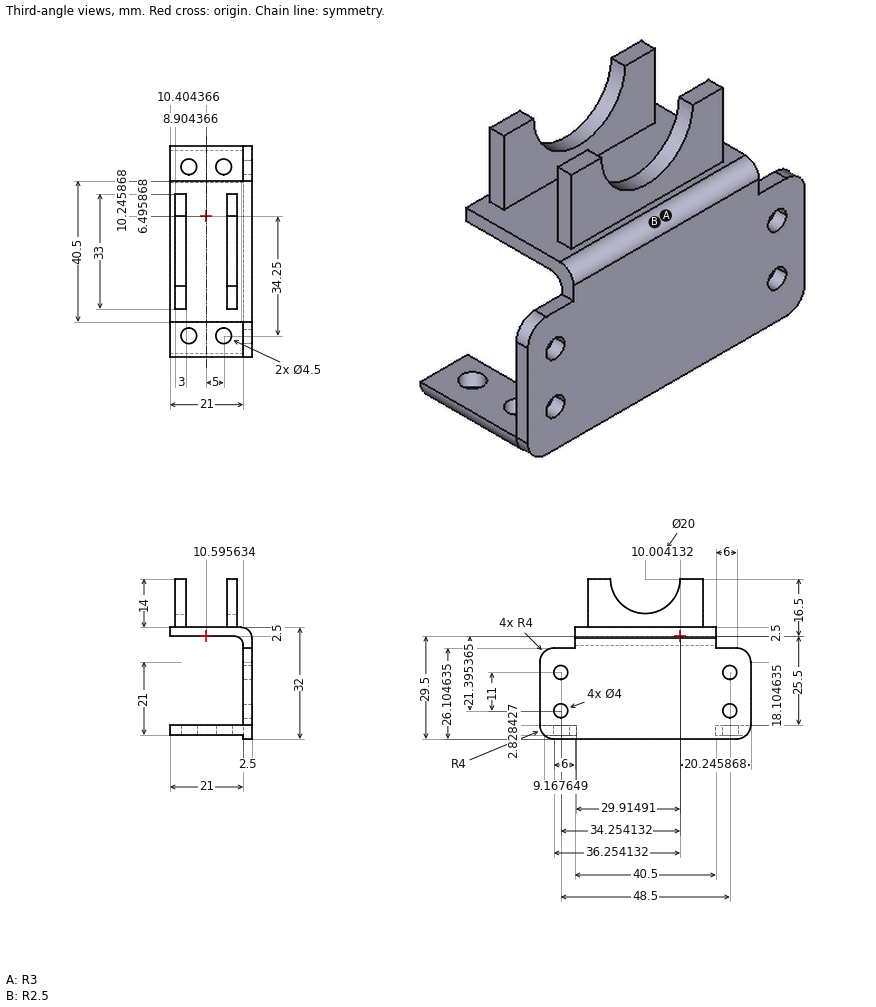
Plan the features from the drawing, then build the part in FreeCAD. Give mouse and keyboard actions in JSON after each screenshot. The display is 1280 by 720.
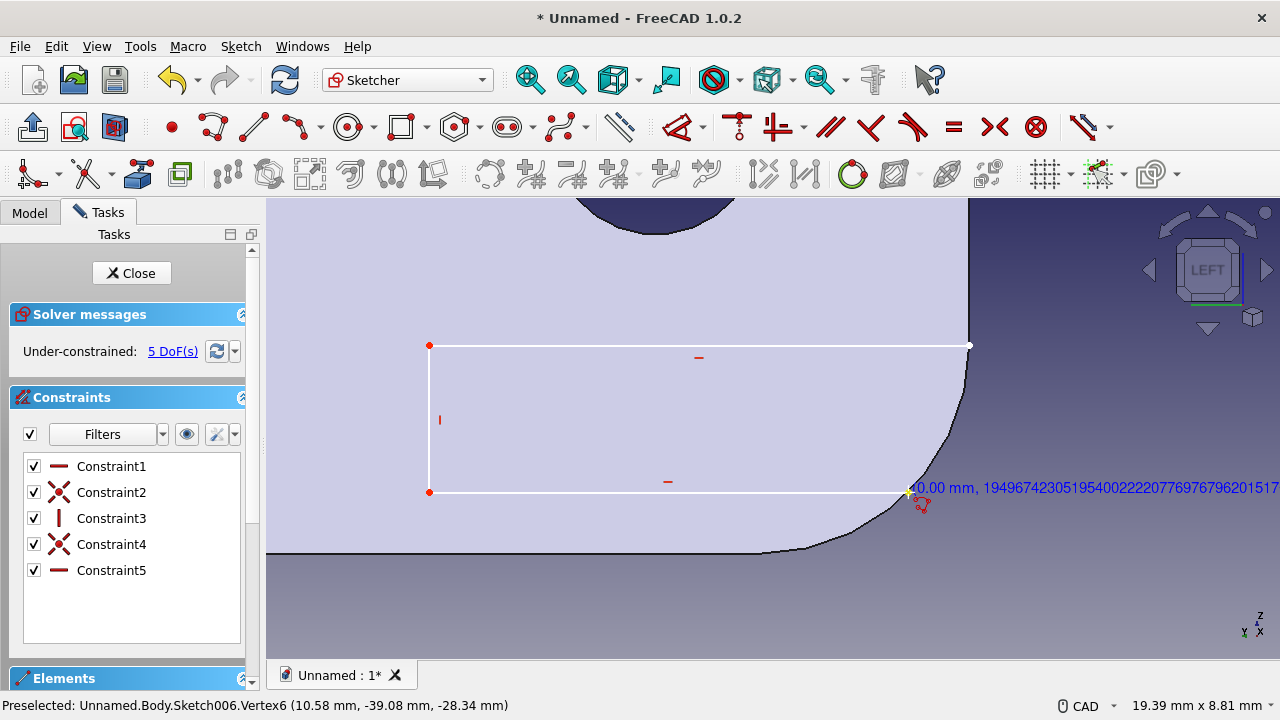
{"action": "left_click", "coordinate": [294, 128]}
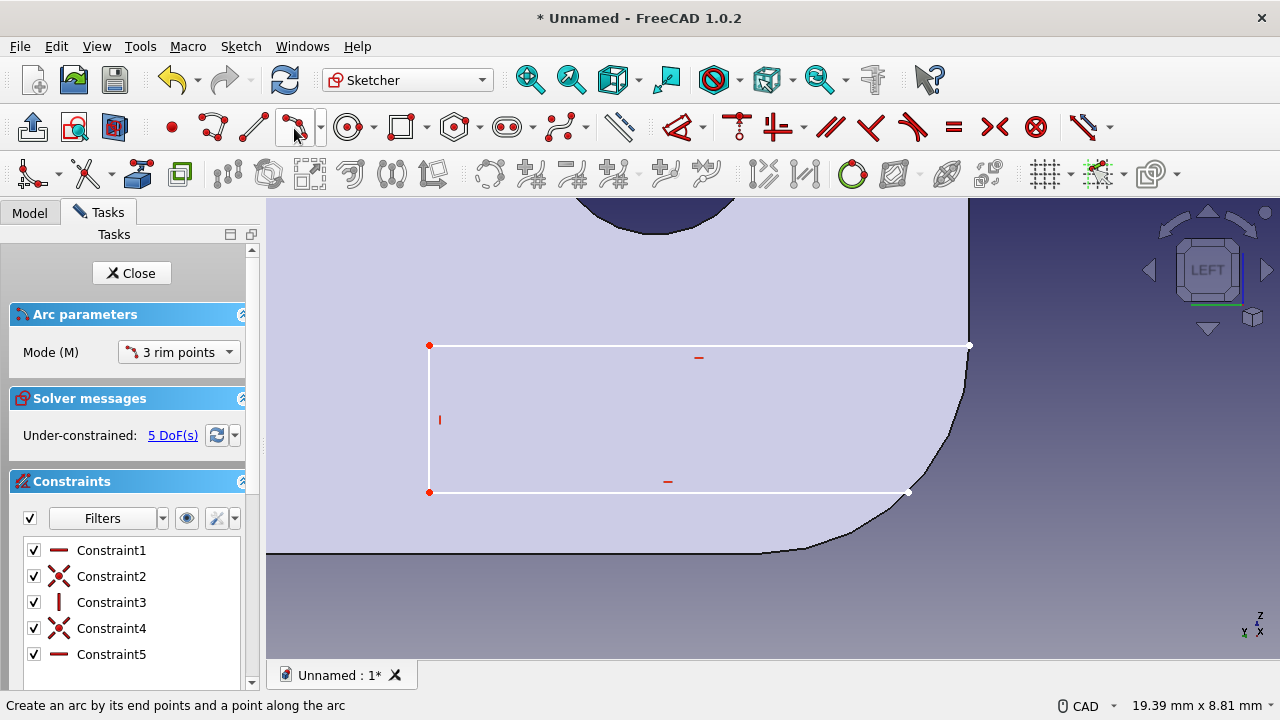
{"action": "left_click", "coordinate": [908, 493]}
{"action": "left_click", "coordinate": [969, 346]}
{"action": "left_click", "coordinate": [953, 425]}
{"action": "key", "text": "Escape"}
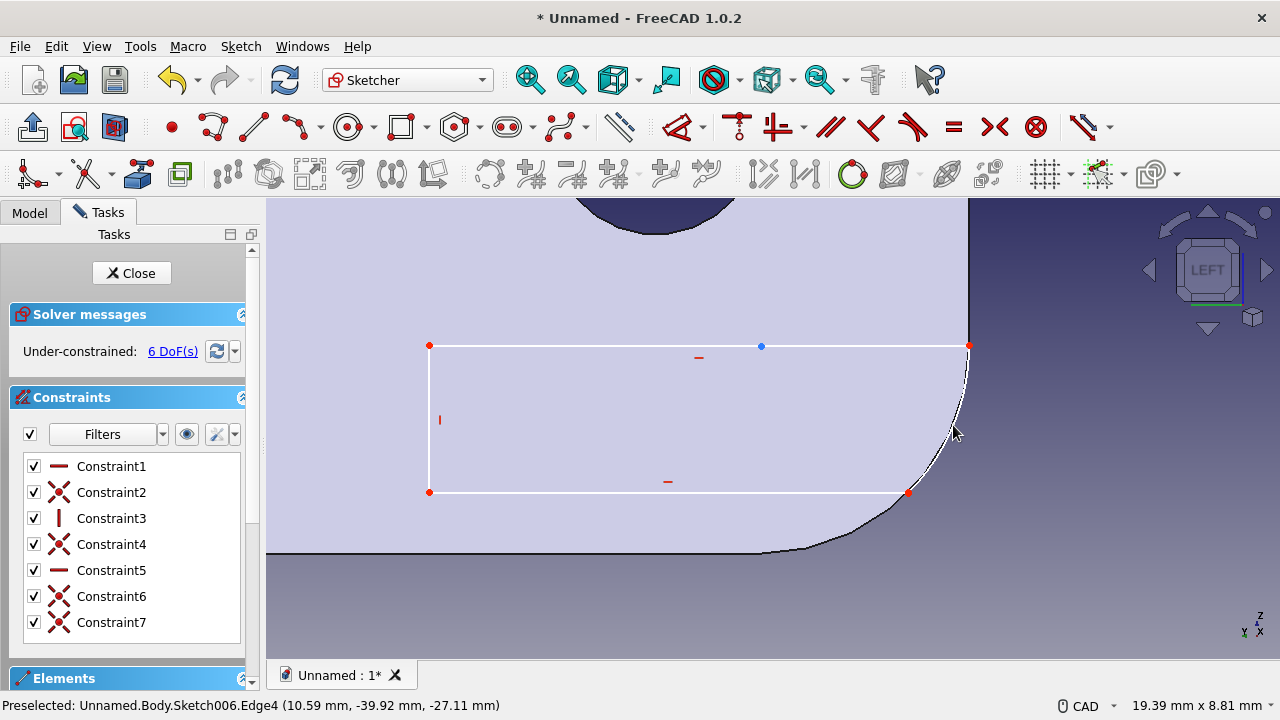
{"action": "left_click", "coordinate": [676, 128]}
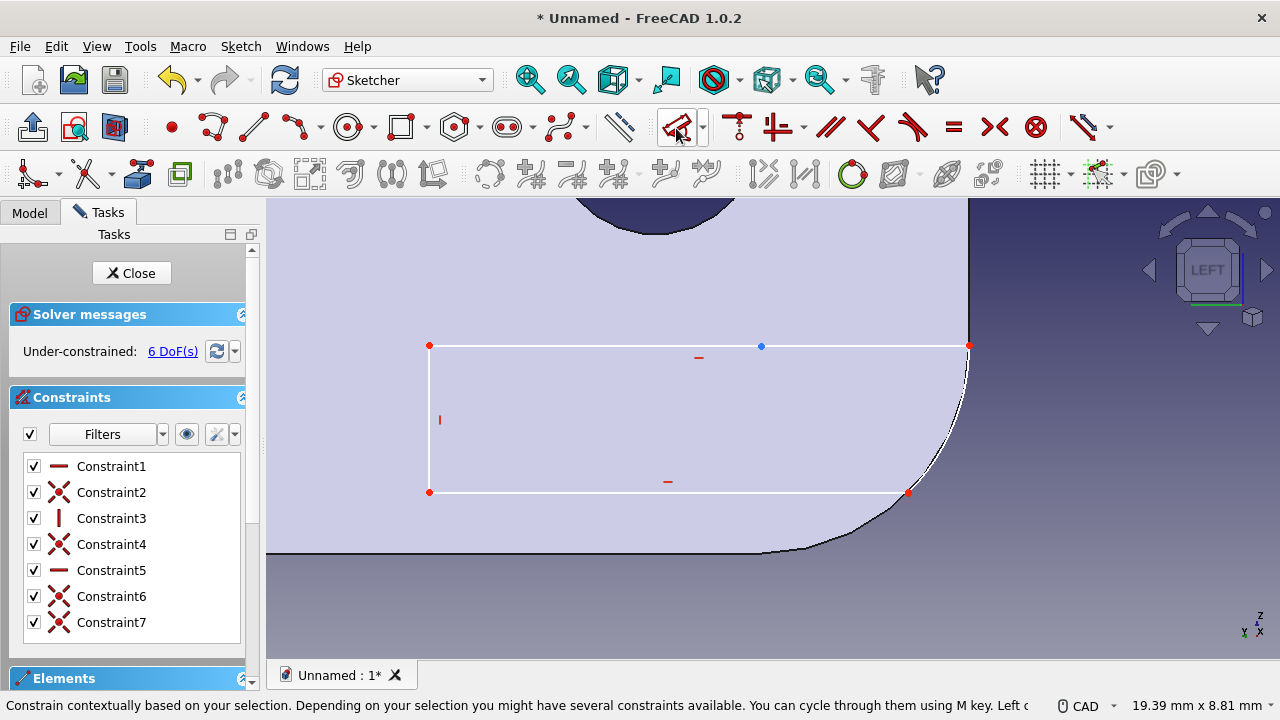
{"action": "left_click", "coordinate": [938, 455]}
{"action": "left_click", "coordinate": [965, 472]}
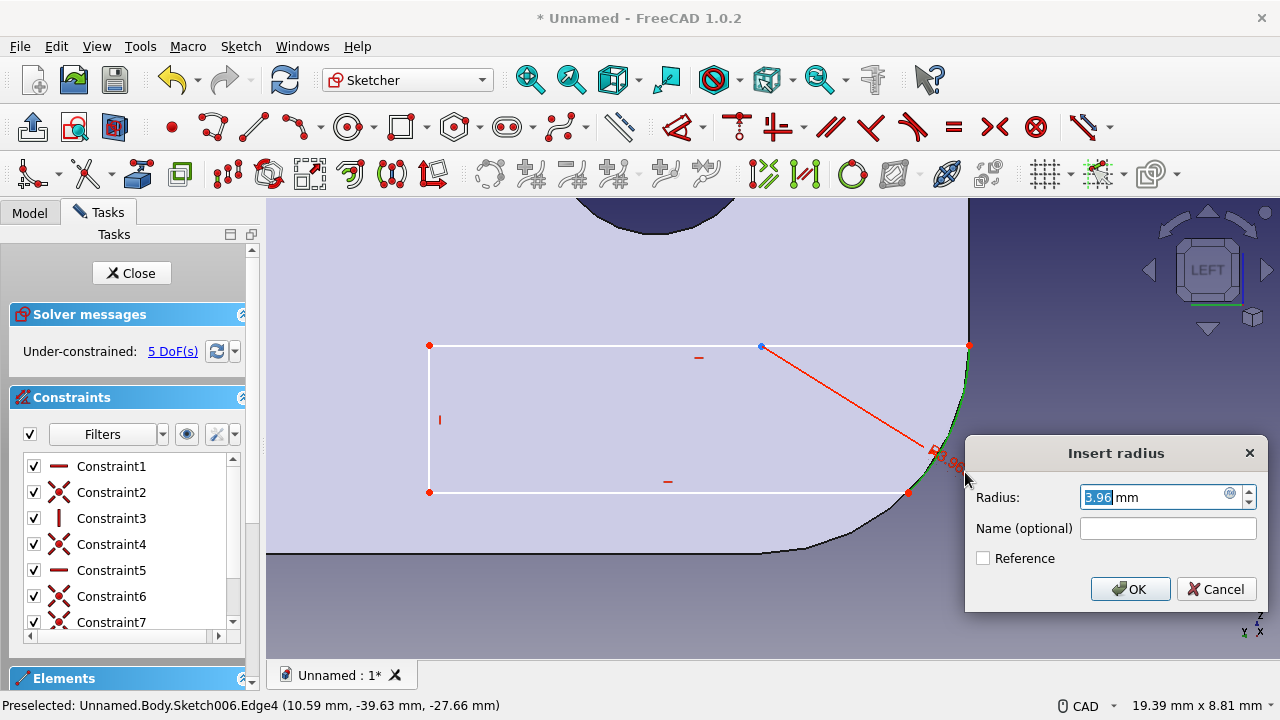
{"action": "type", "text": "4"}
{"action": "key", "text": "Return"}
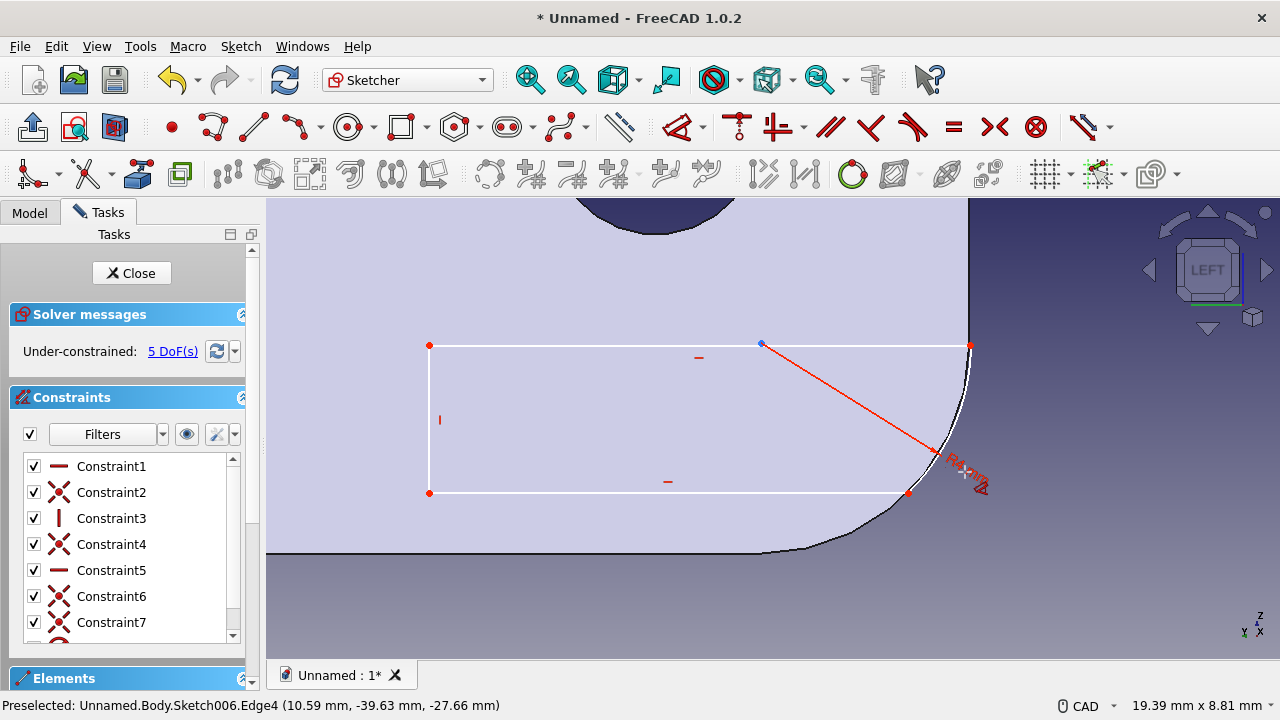
{"action": "left_click", "coordinate": [971, 346]}
{"action": "left_click", "coordinate": [1005, 286]}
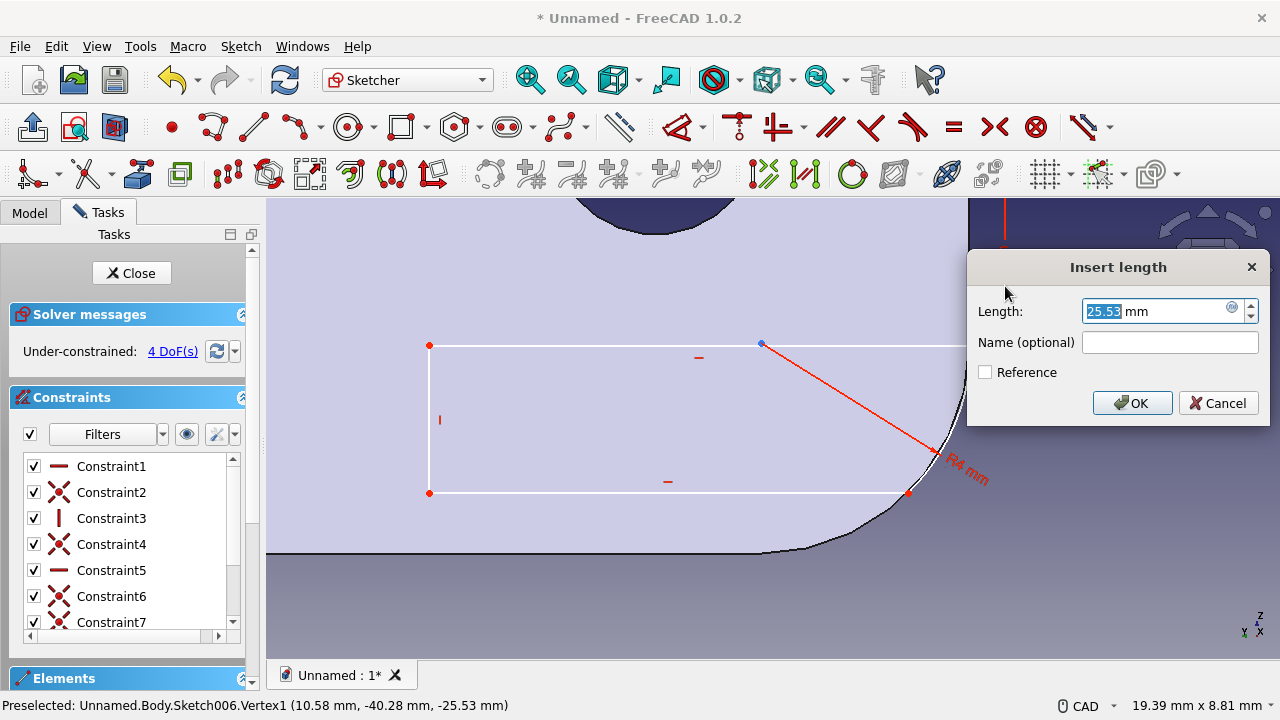
{"action": "type", "text": "25.5"}
{"action": "key", "text": "Return"}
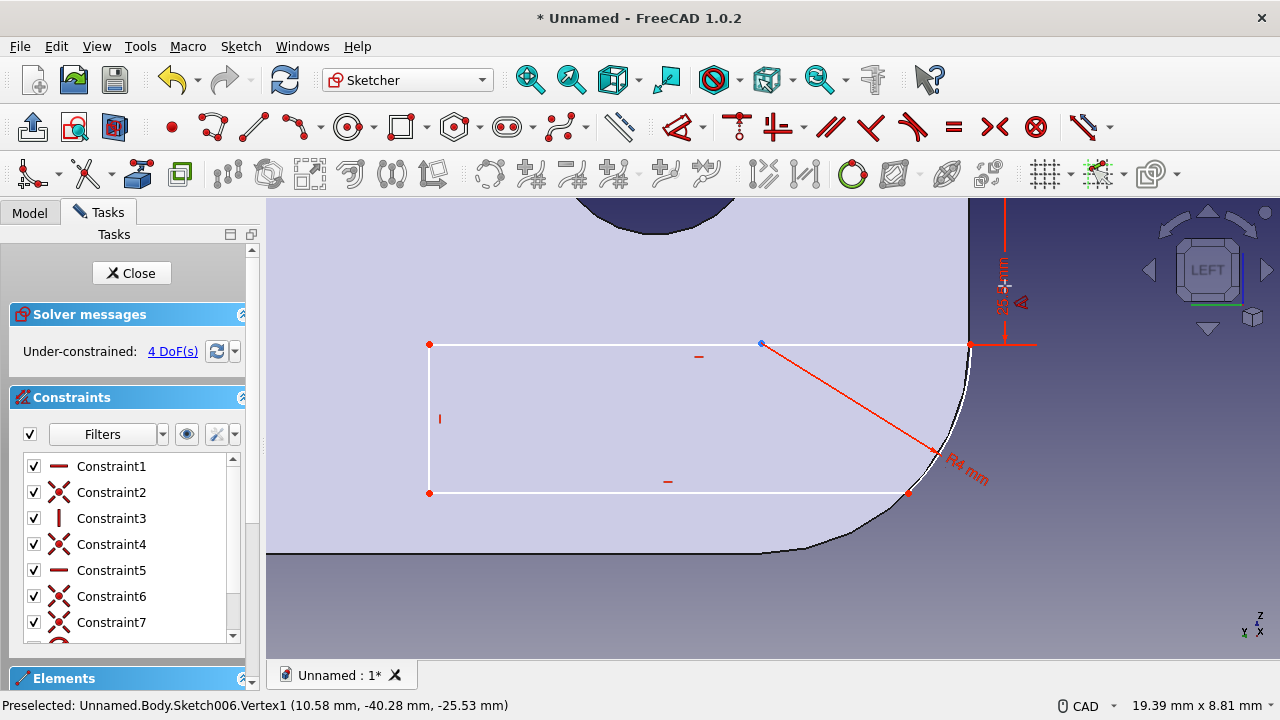
{"action": "left_click", "coordinate": [762, 343]}
{"action": "left_click", "coordinate": [796, 285]}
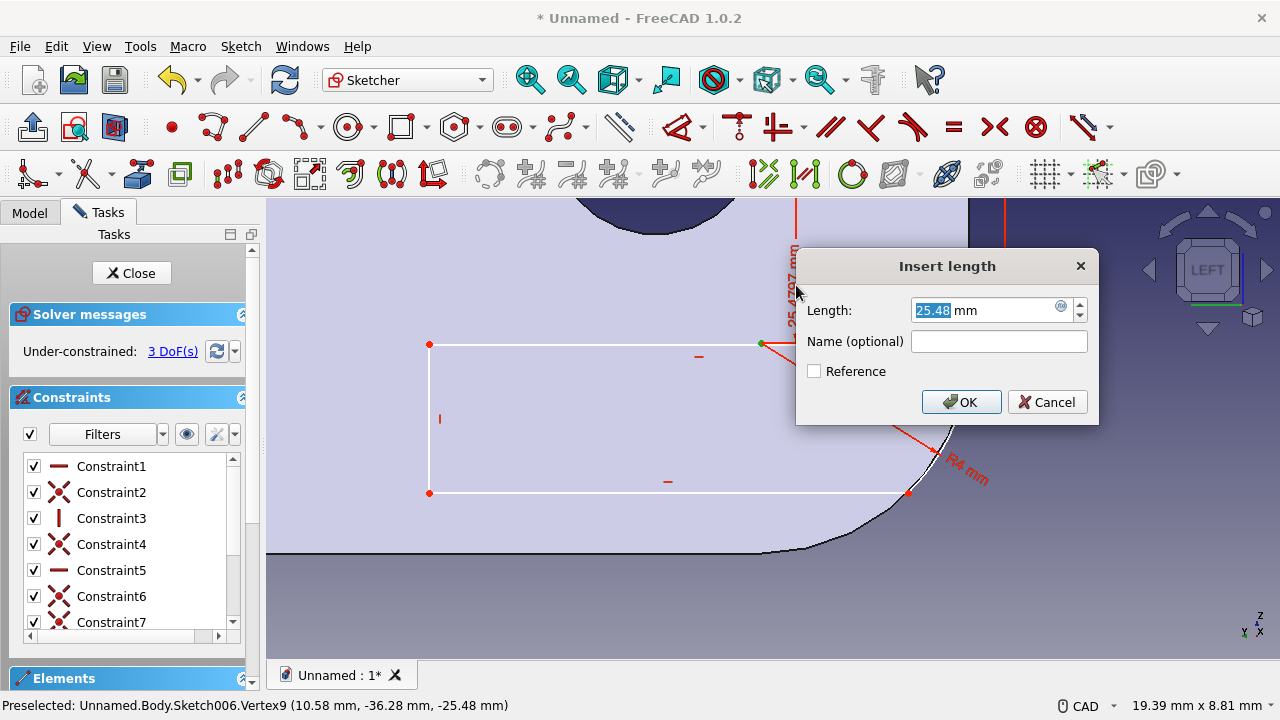
{"action": "type", "text": "25.5"}
{"action": "key", "text": "Return"}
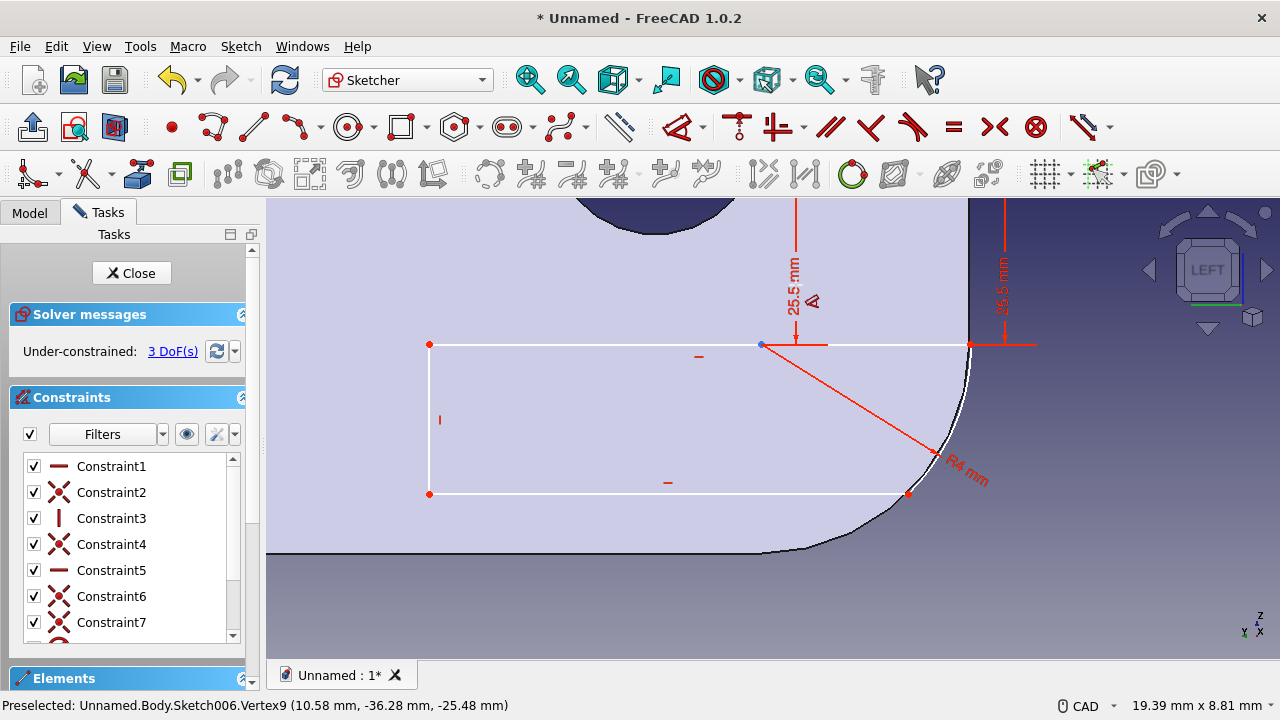
{"action": "left_click", "coordinate": [429, 389]}
{"action": "left_click", "coordinate": [395, 419]}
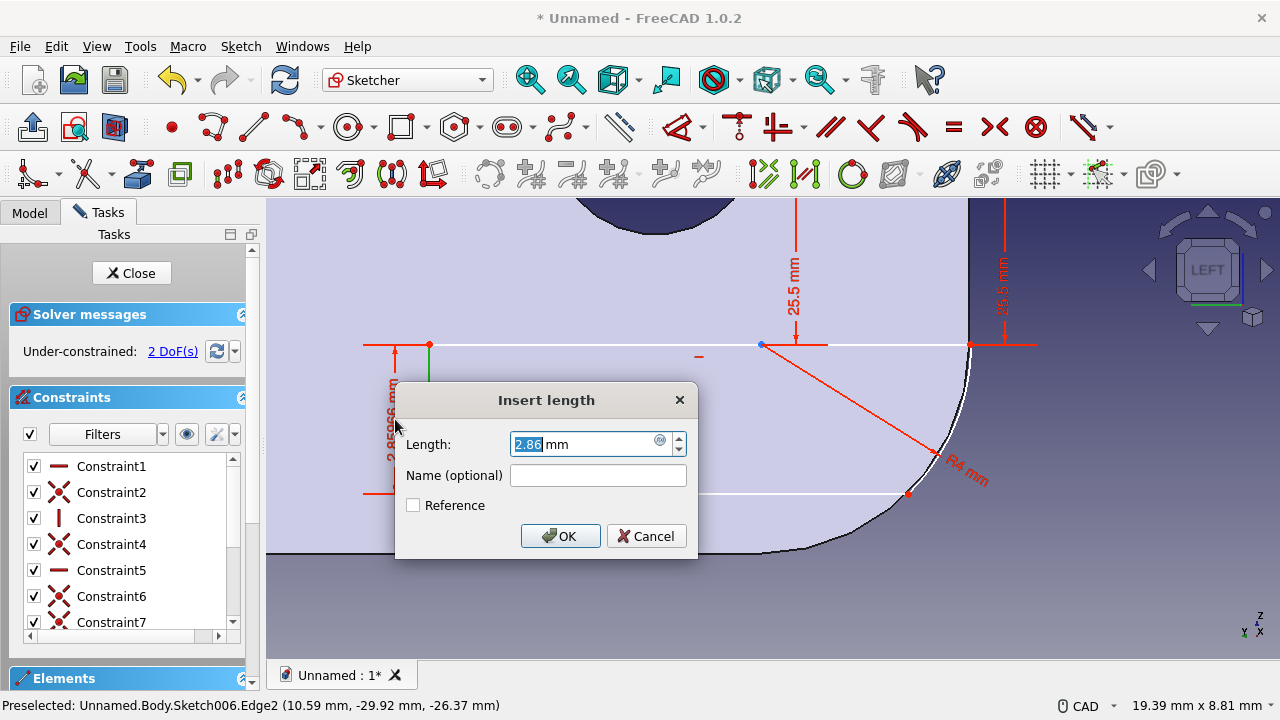
{"action": "type", "text": "2.828427"}
{"action": "key", "text": "Return"}